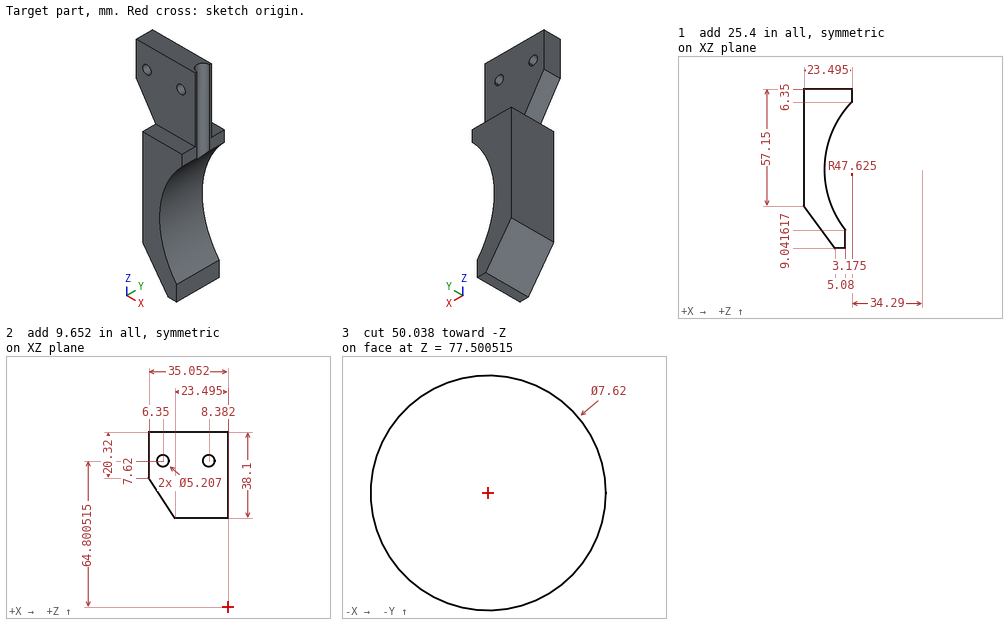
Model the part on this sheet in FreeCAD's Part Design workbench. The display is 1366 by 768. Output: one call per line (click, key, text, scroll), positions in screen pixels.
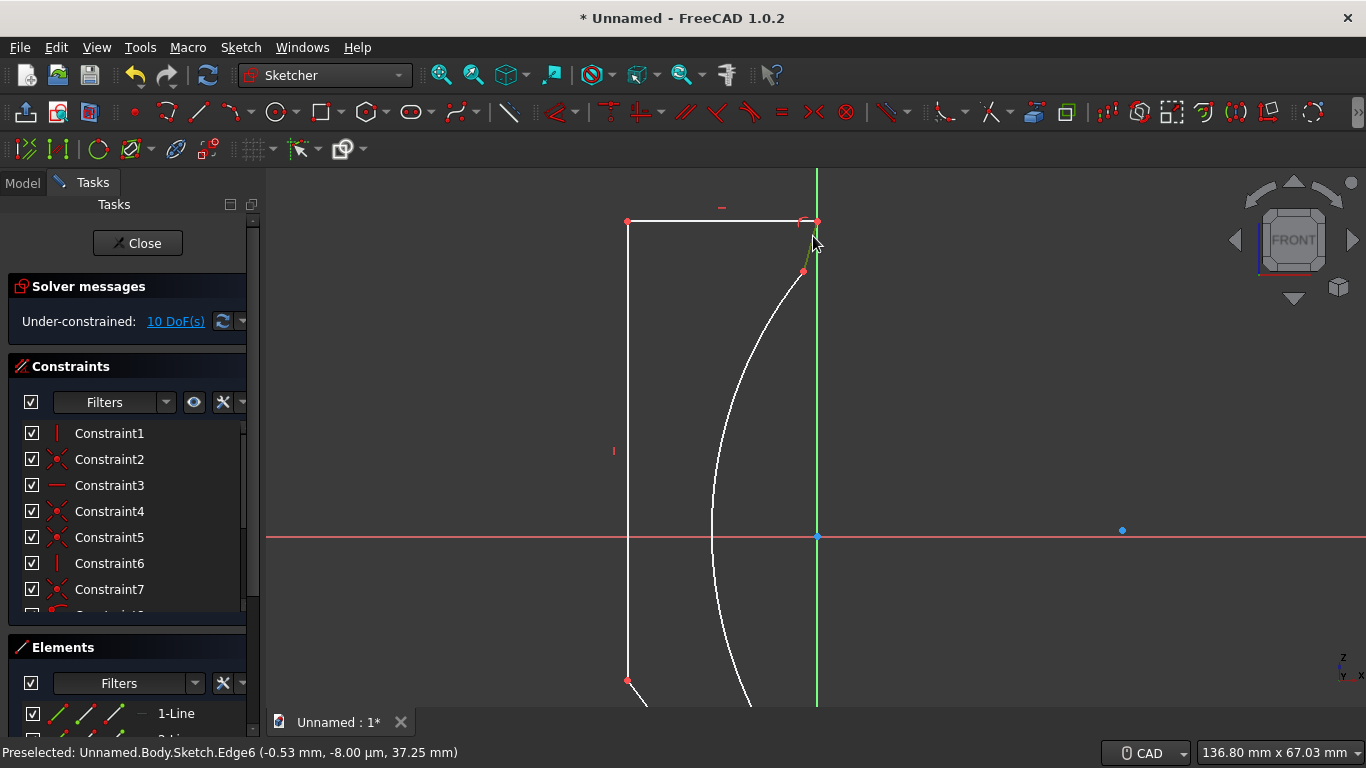
click(664, 112)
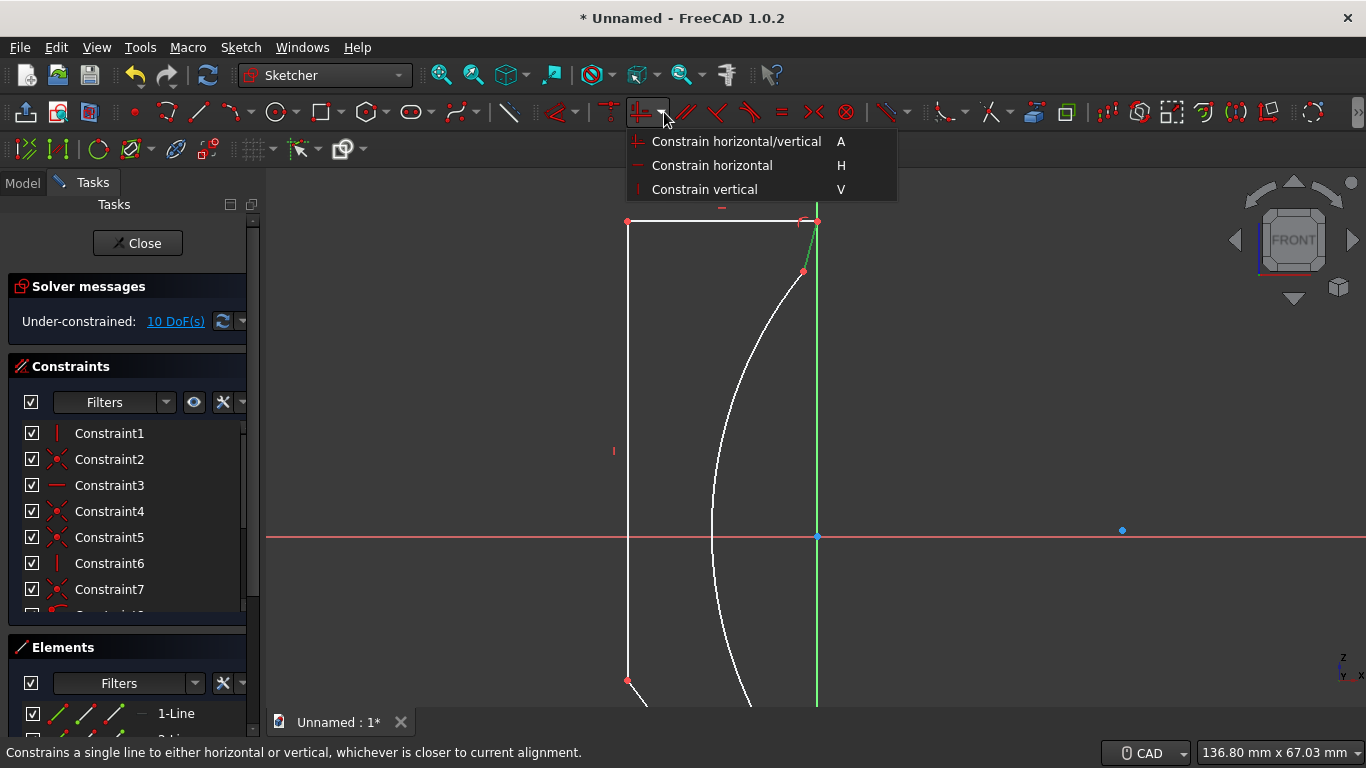
click(762, 189)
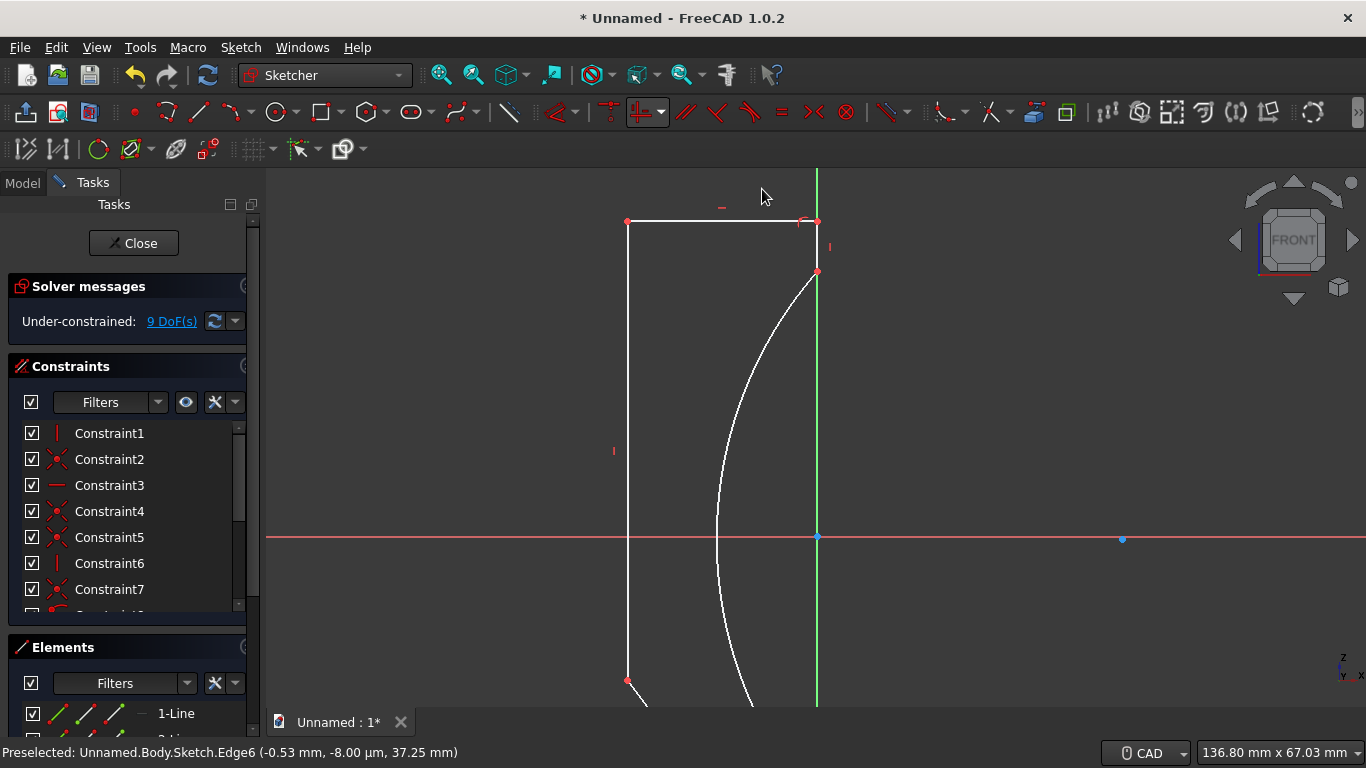
click(1123, 539)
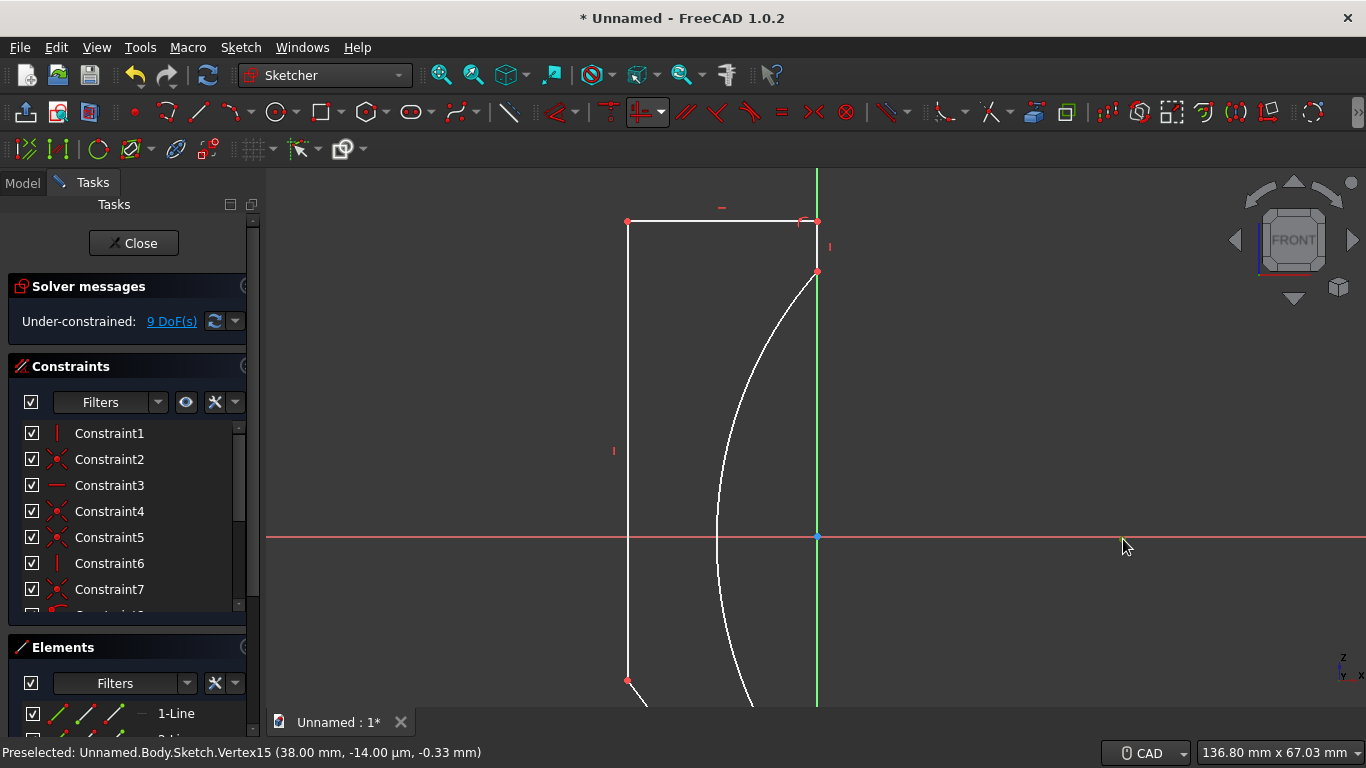
click(359, 537)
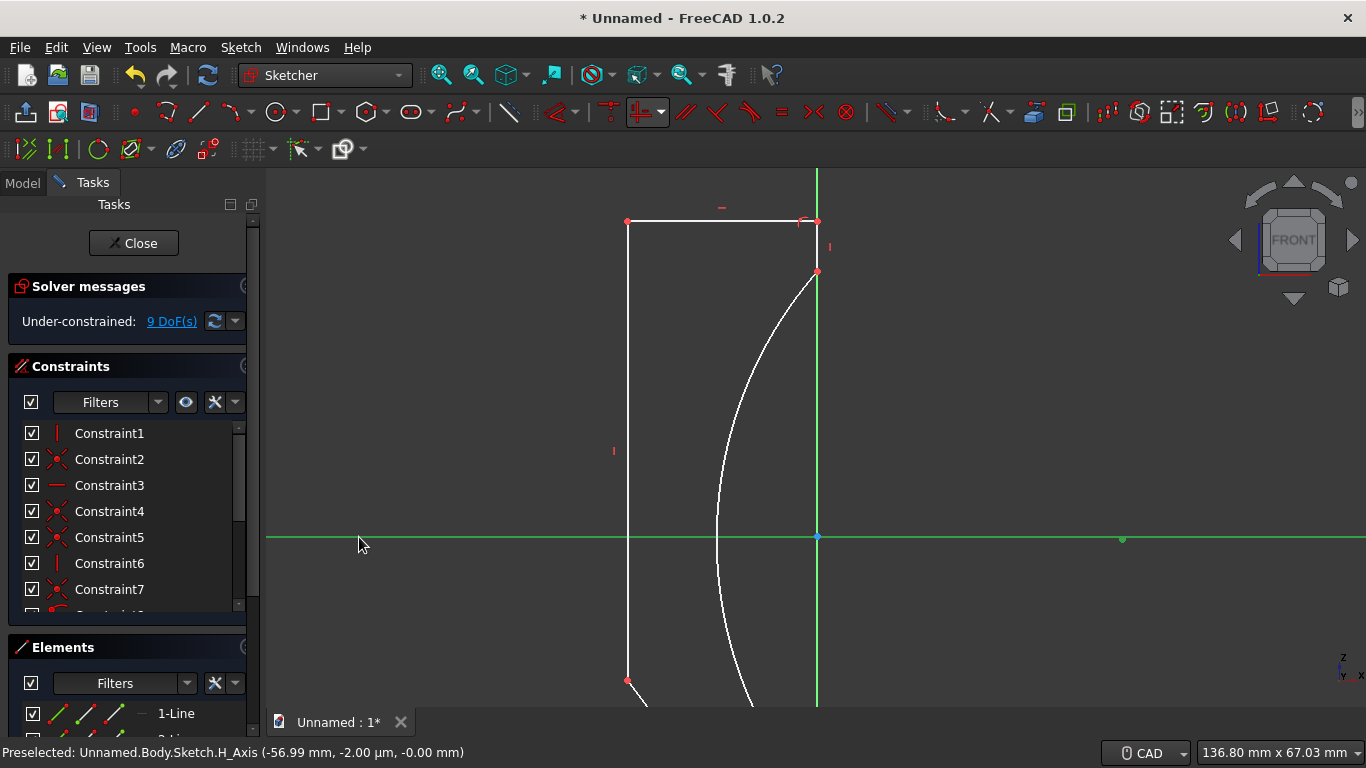
click(610, 112)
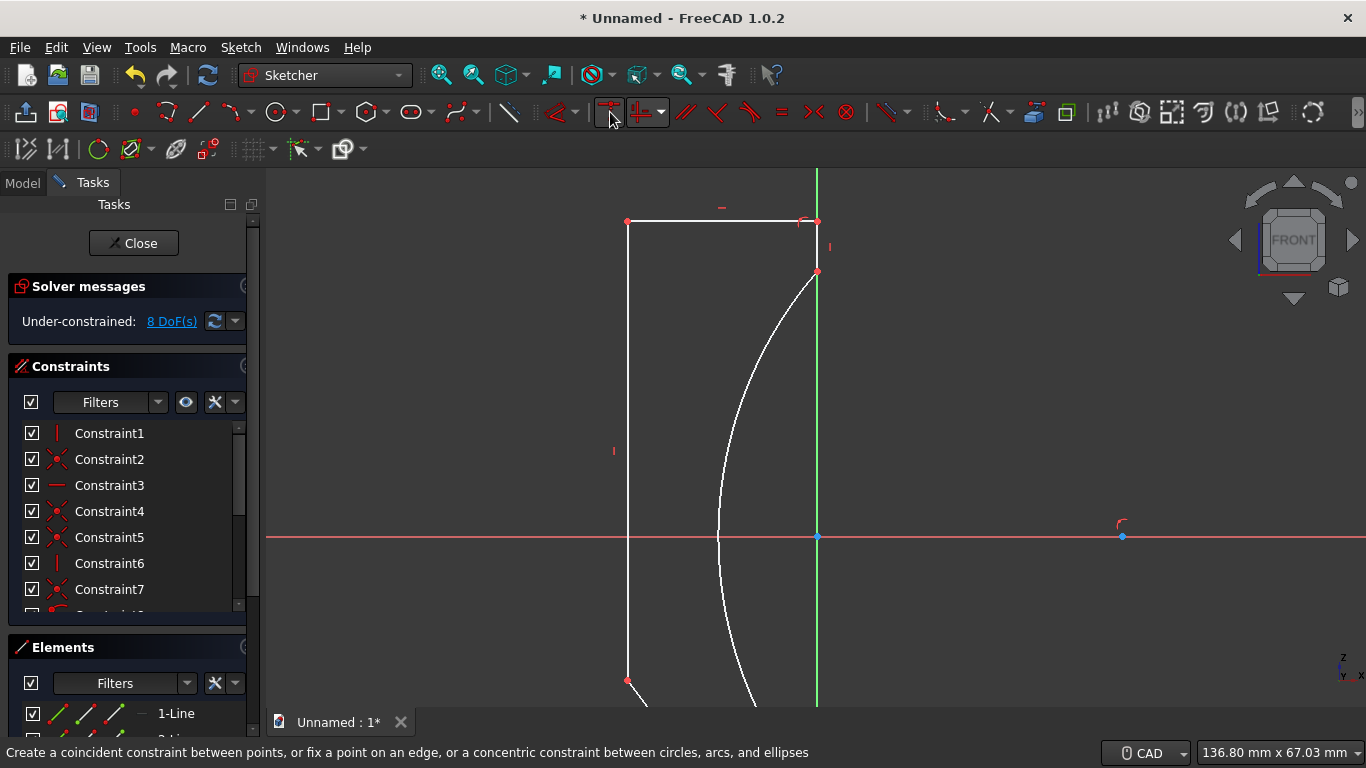
click(738, 413)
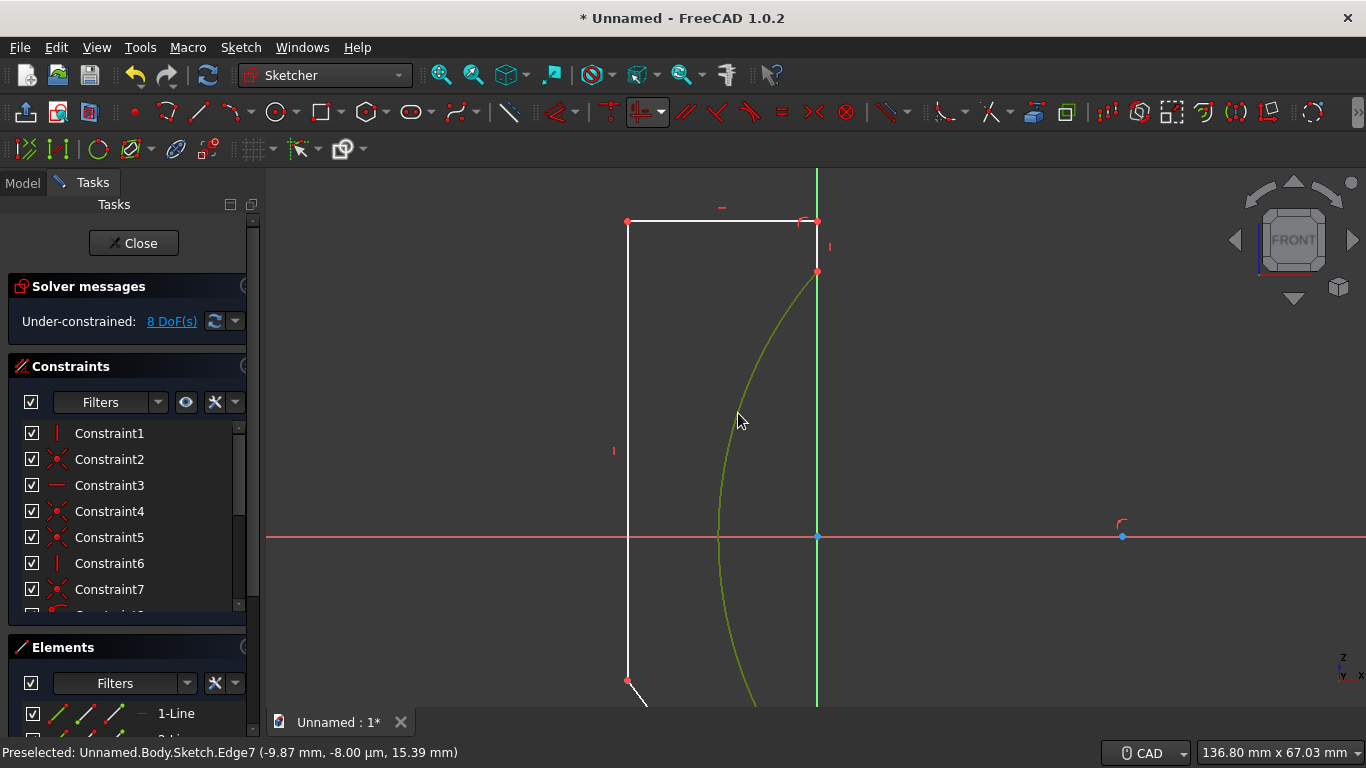
click(578, 112)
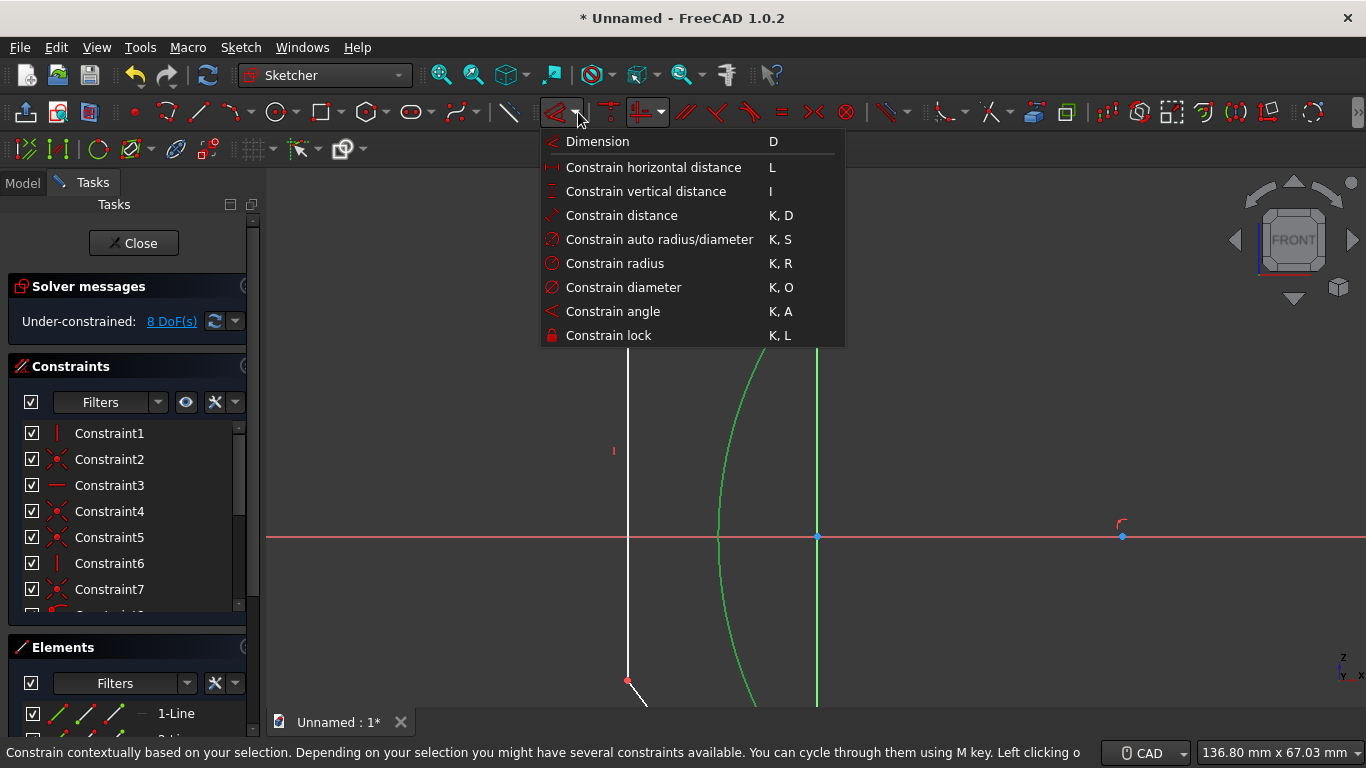
click(693, 263)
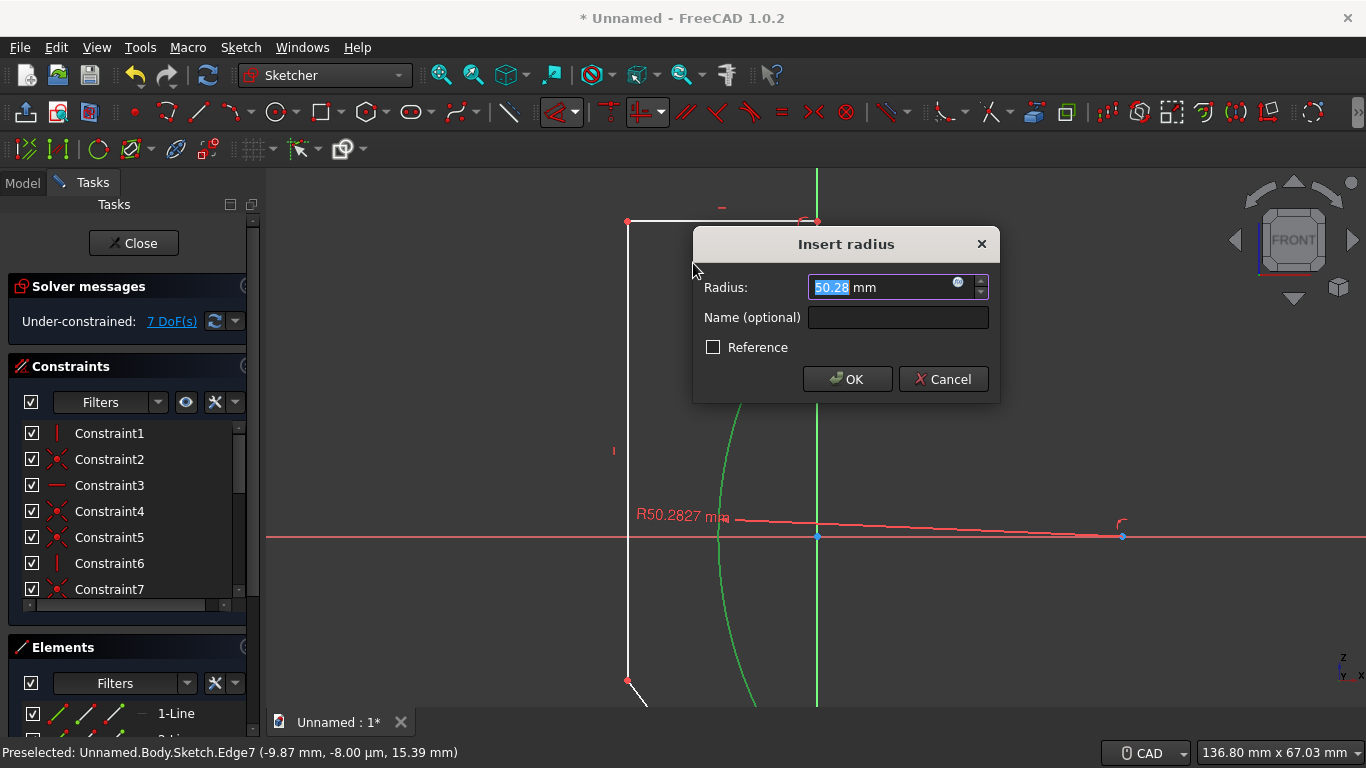
text(47.625)
key(Return)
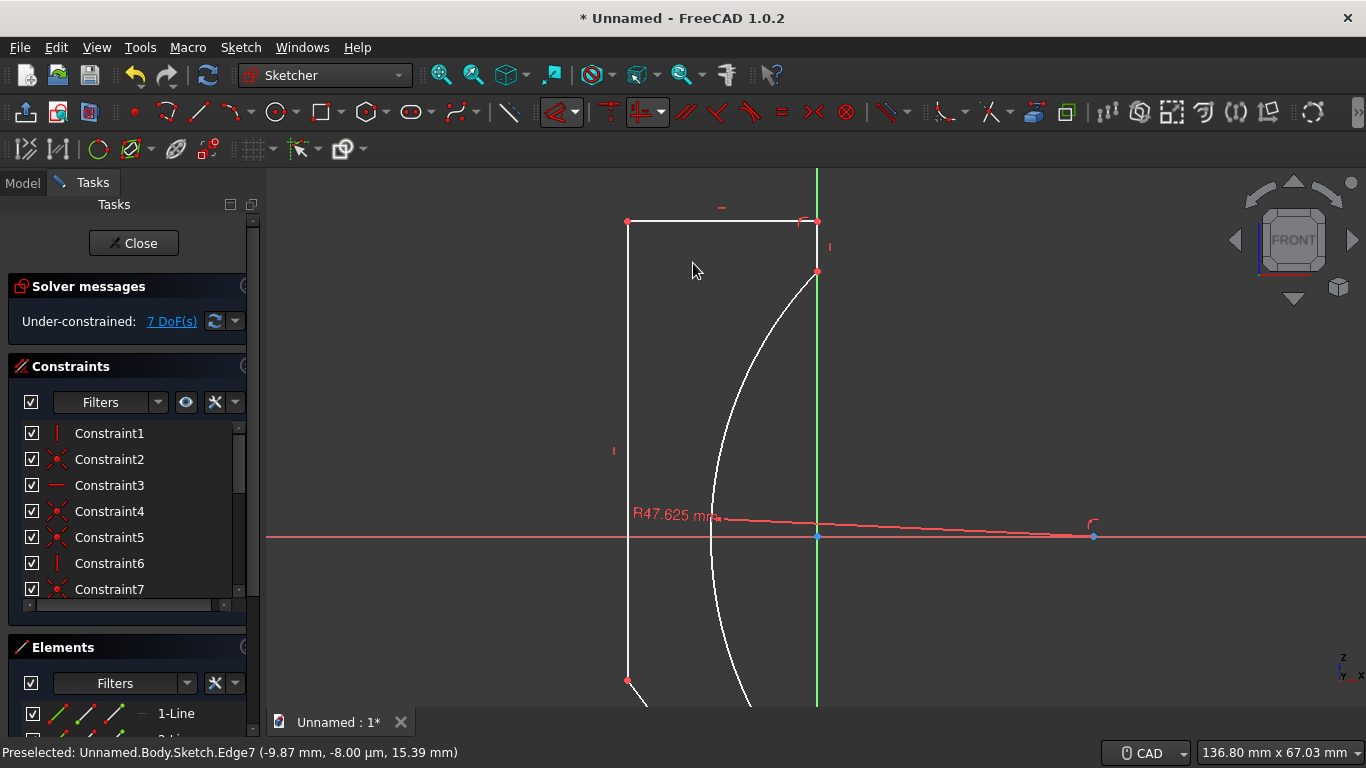
scroll(778, 322, down, 3)